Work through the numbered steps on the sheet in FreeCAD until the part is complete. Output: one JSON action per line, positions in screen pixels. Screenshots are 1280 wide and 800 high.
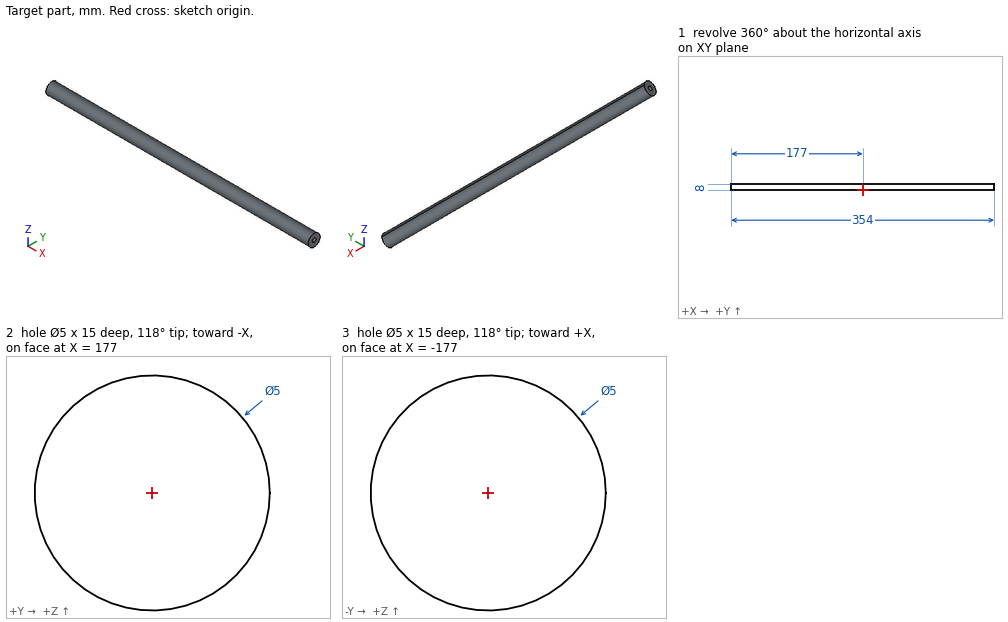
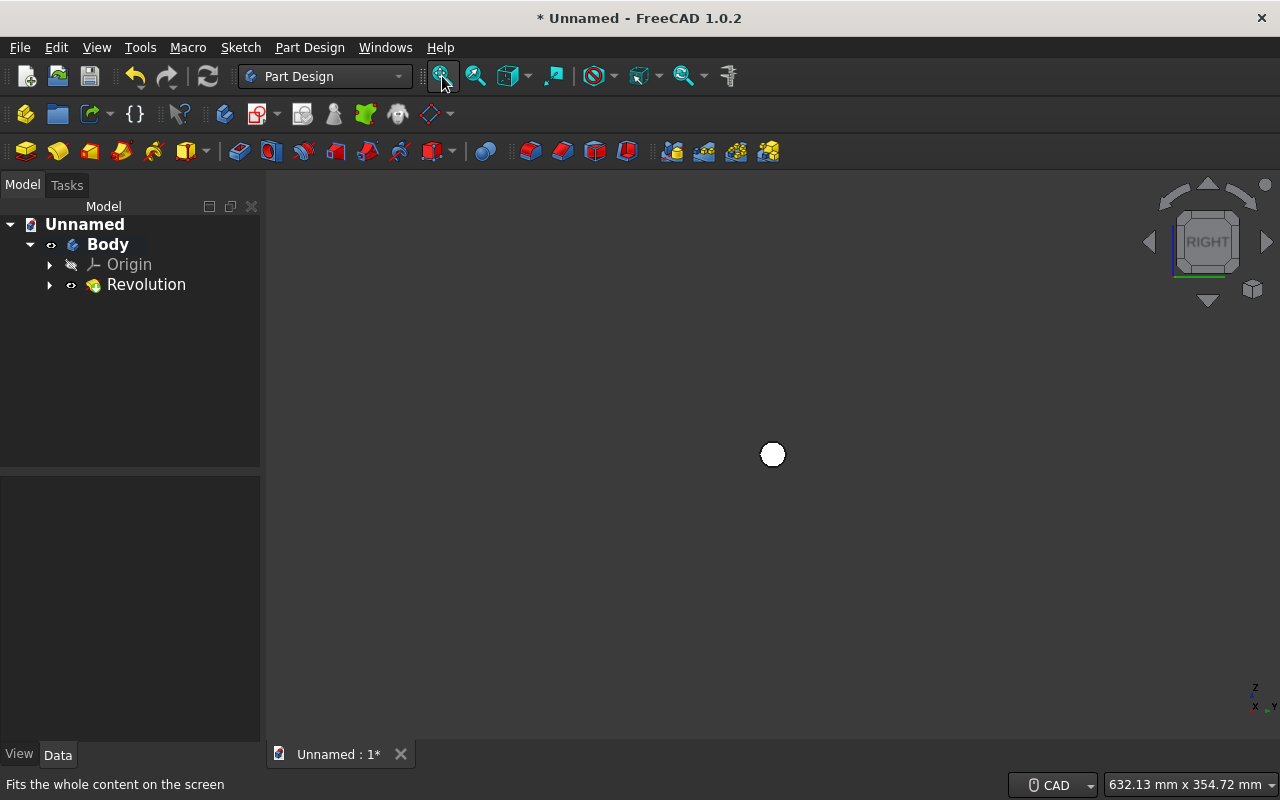
{"action": "left_click", "coordinate": [773, 453]}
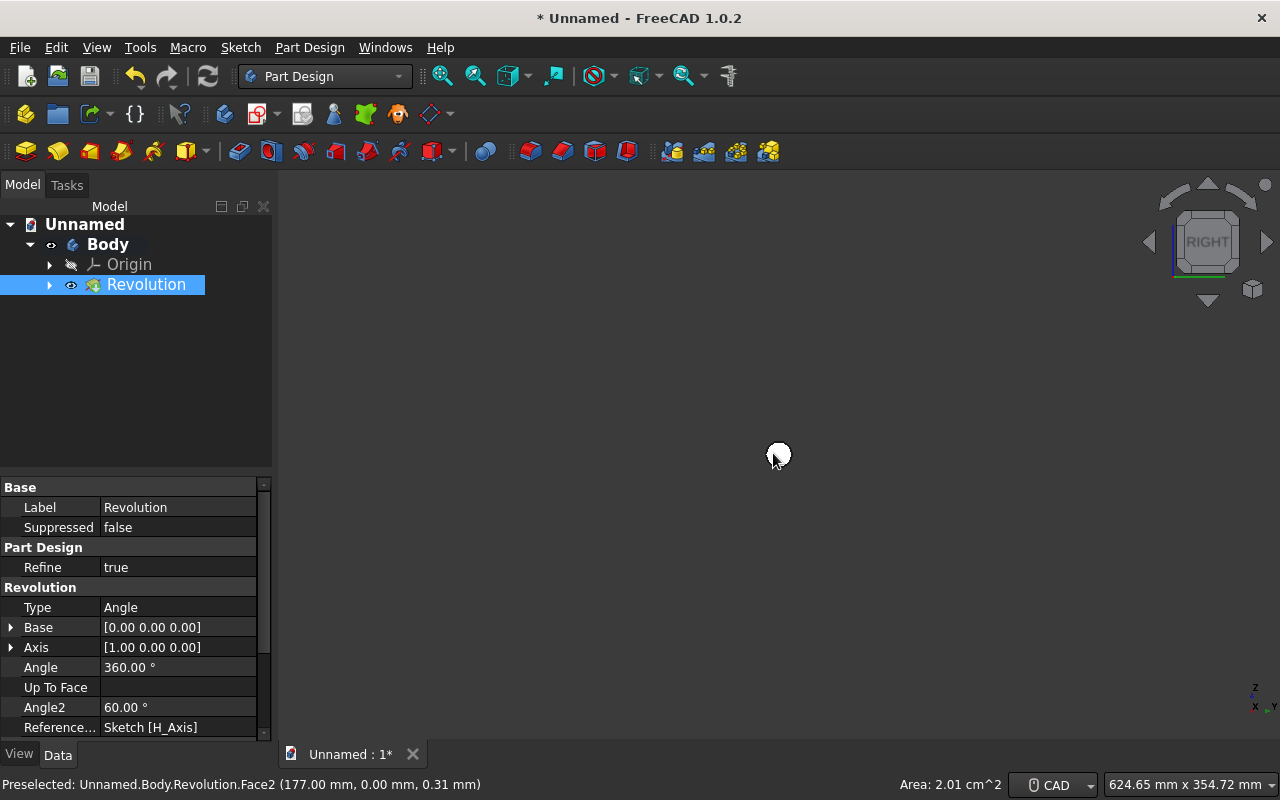
{"action": "left_click", "coordinate": [258, 114]}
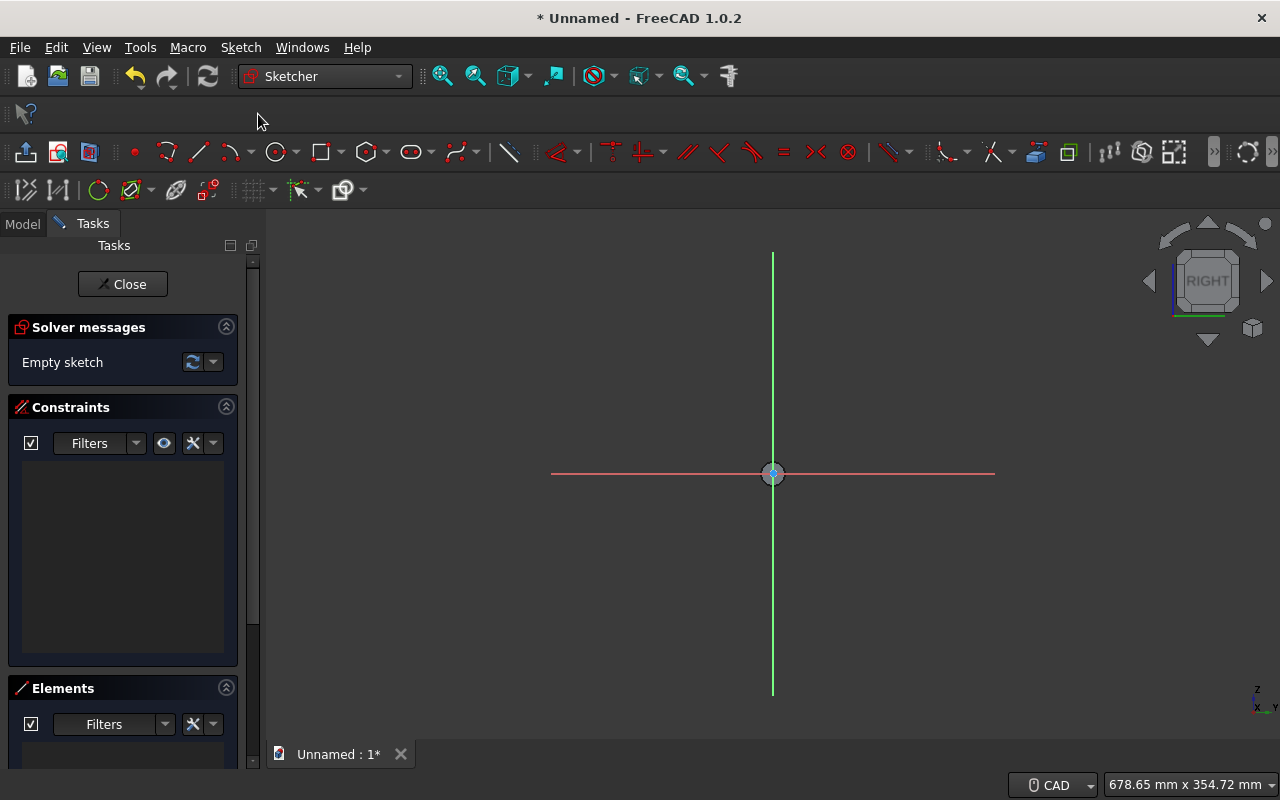
{"action": "scroll", "coordinate": [777, 474], "scroll_direction": "up", "scroll_amount": 15}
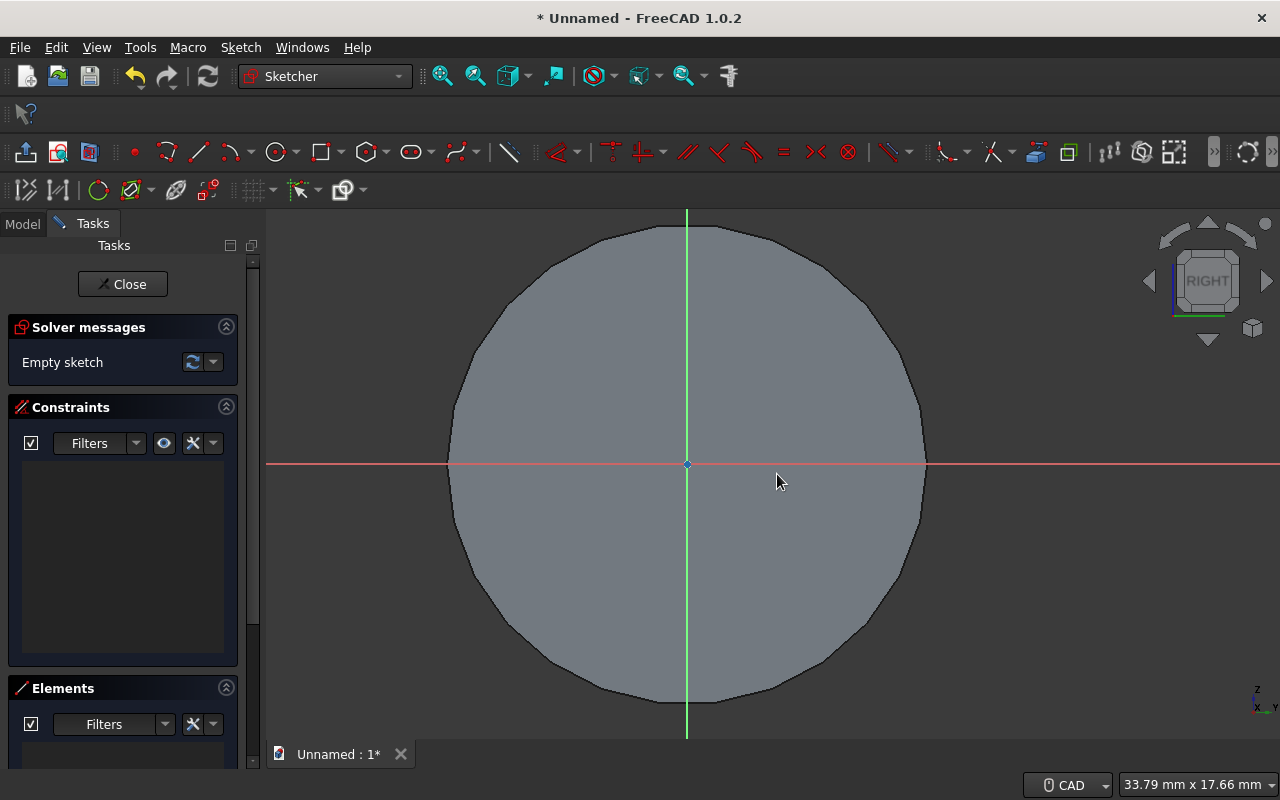
{"action": "scroll", "coordinate": [673, 457], "scroll_direction": "up", "scroll_amount": 4}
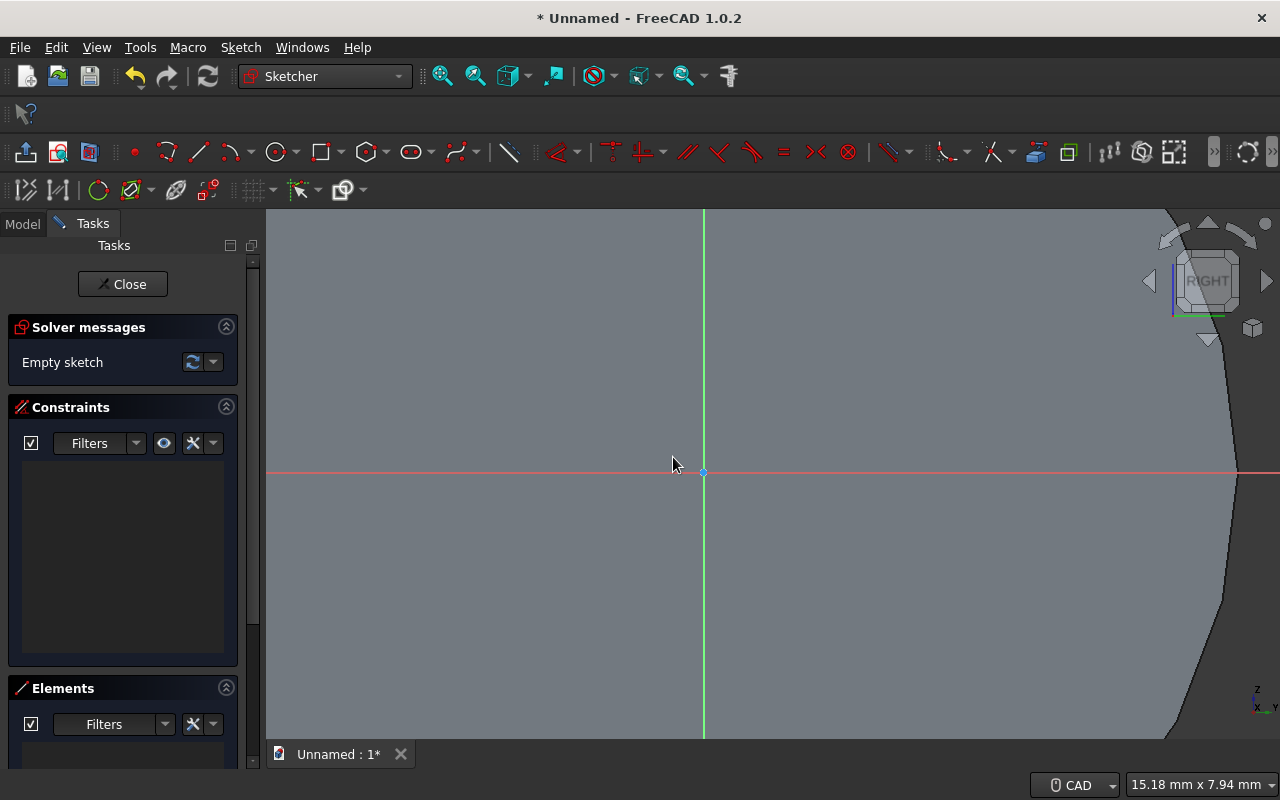
{"action": "key", "text": "g c"}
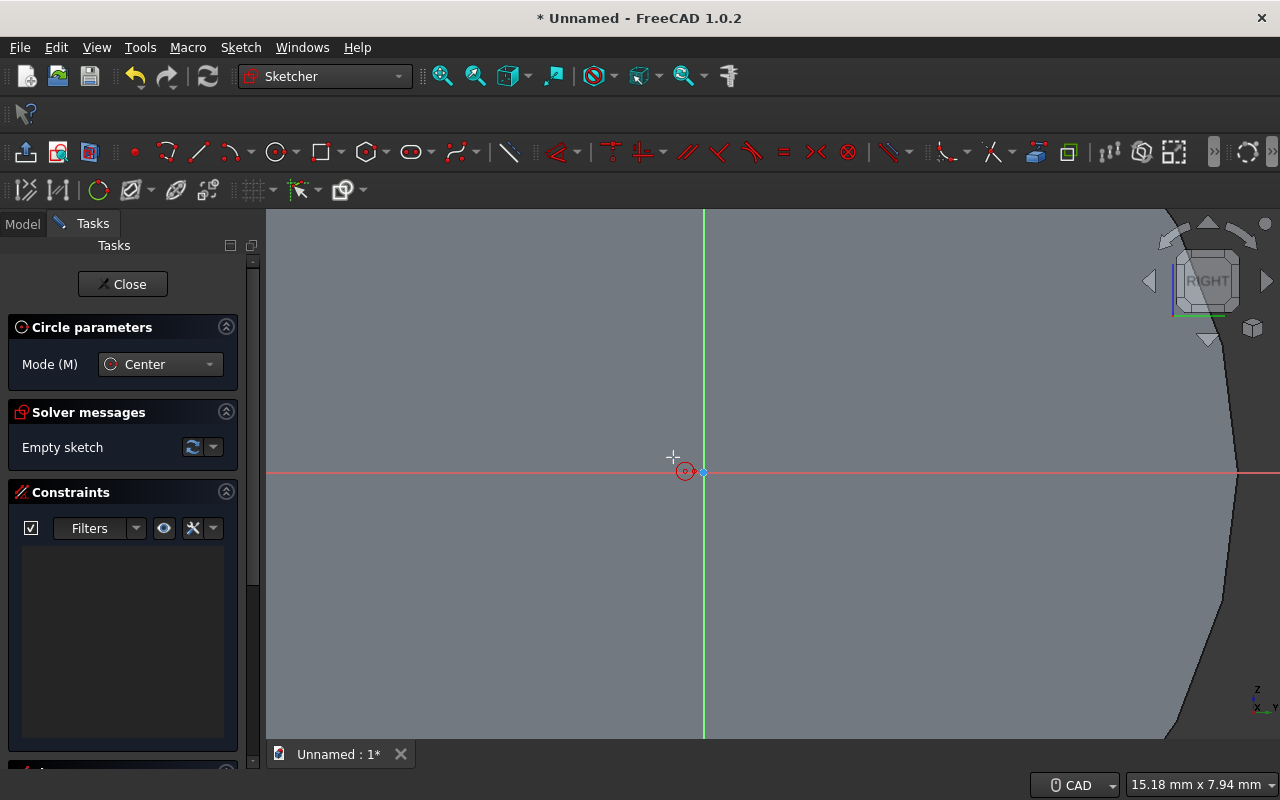
{"action": "left_click", "coordinate": [704, 473]}
{"action": "left_click", "coordinate": [822, 355]}
{"action": "key", "text": "Escape"}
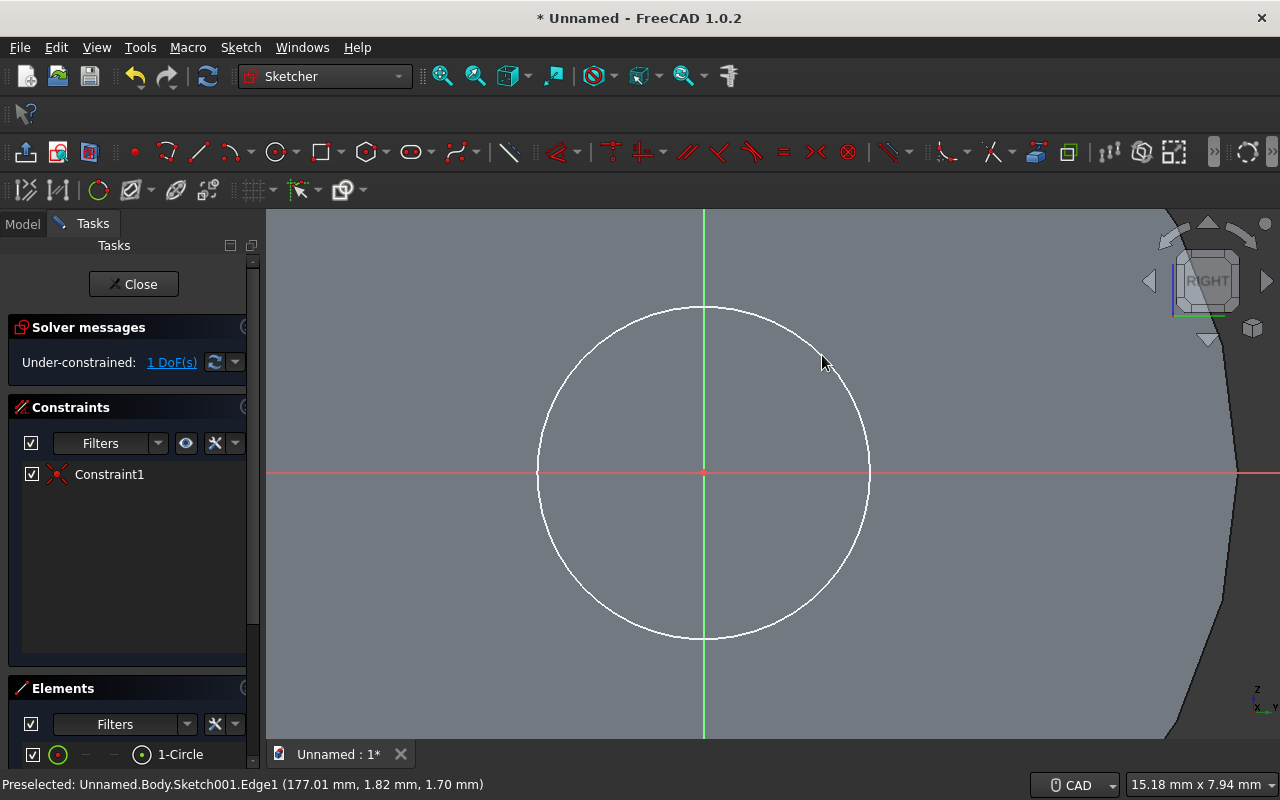
{"action": "left_click", "coordinate": [556, 152]}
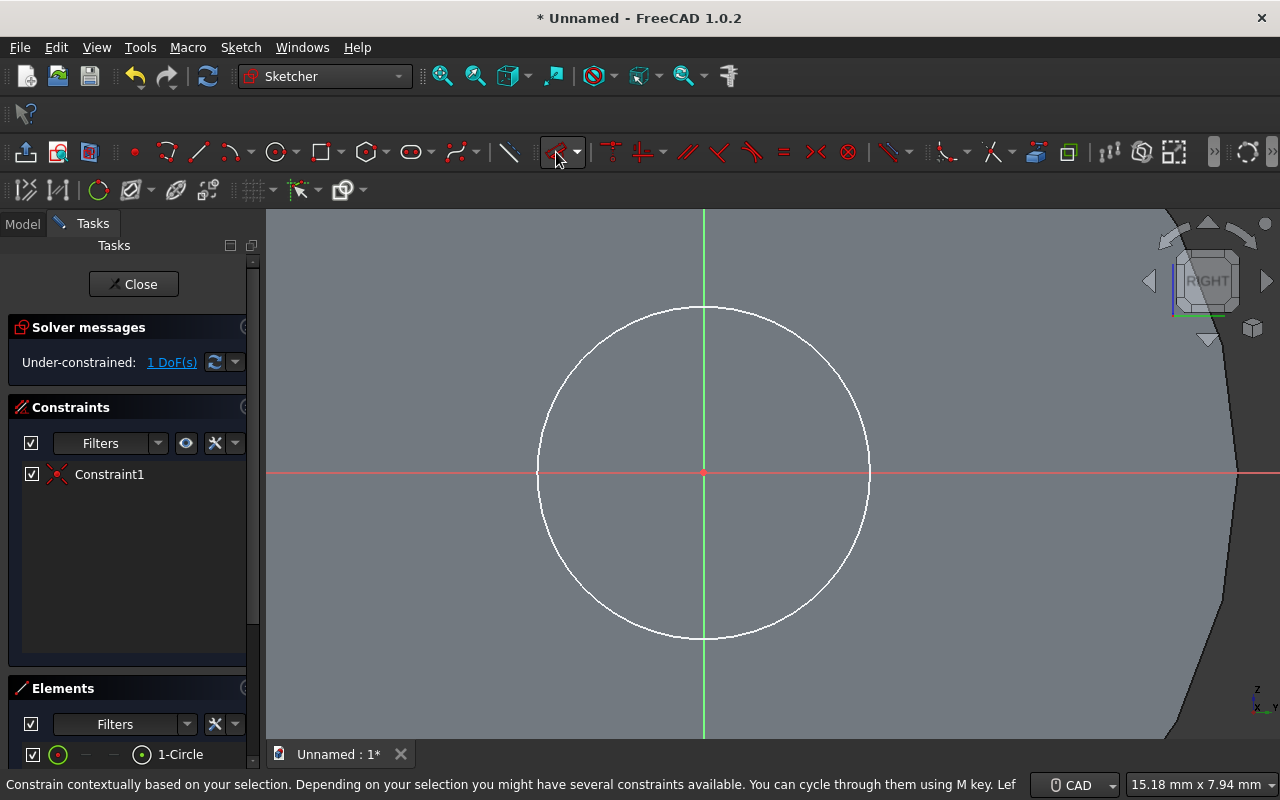
{"action": "left_click", "coordinate": [821, 355]}
{"action": "left_click", "coordinate": [844, 332]}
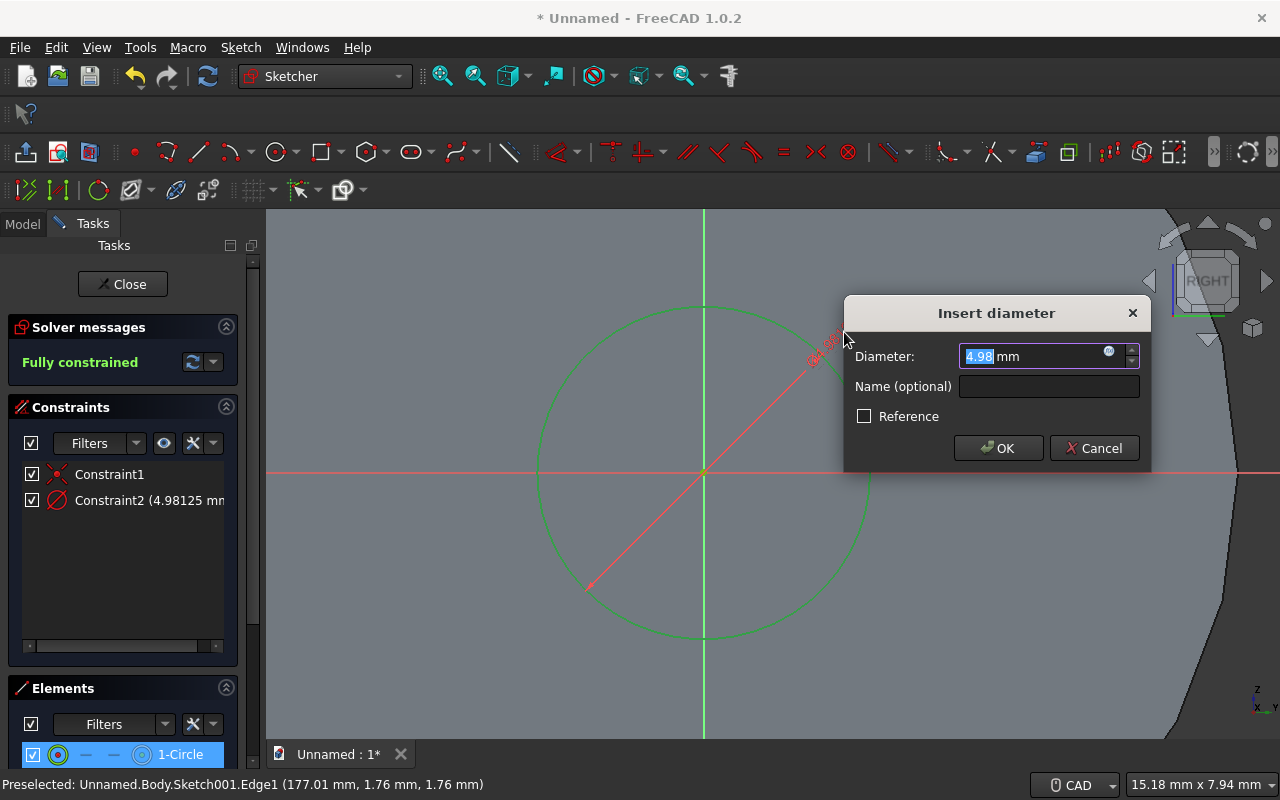
{"action": "type", "text": "5"}
{"action": "key", "text": "Return"}
{"action": "key", "text": "Escape"}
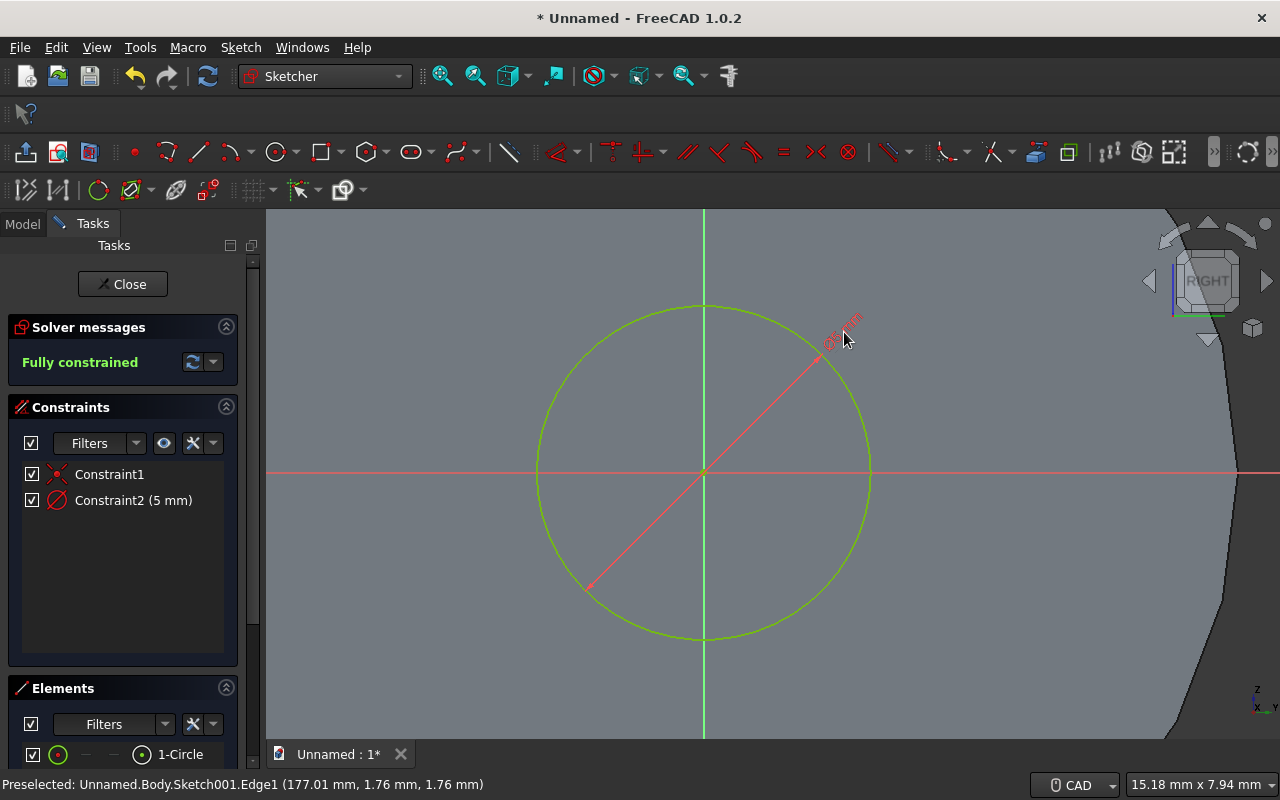
{"action": "left_click", "coordinate": [123, 284]}